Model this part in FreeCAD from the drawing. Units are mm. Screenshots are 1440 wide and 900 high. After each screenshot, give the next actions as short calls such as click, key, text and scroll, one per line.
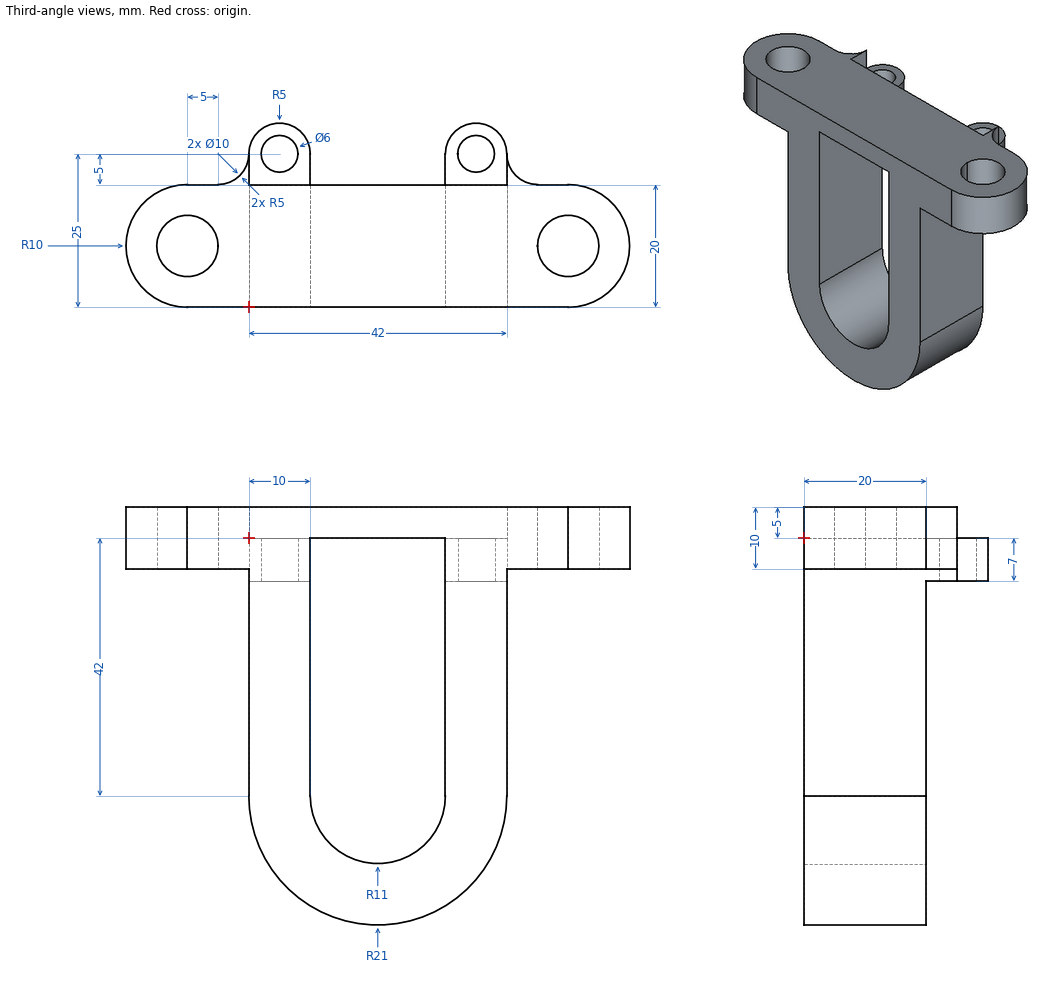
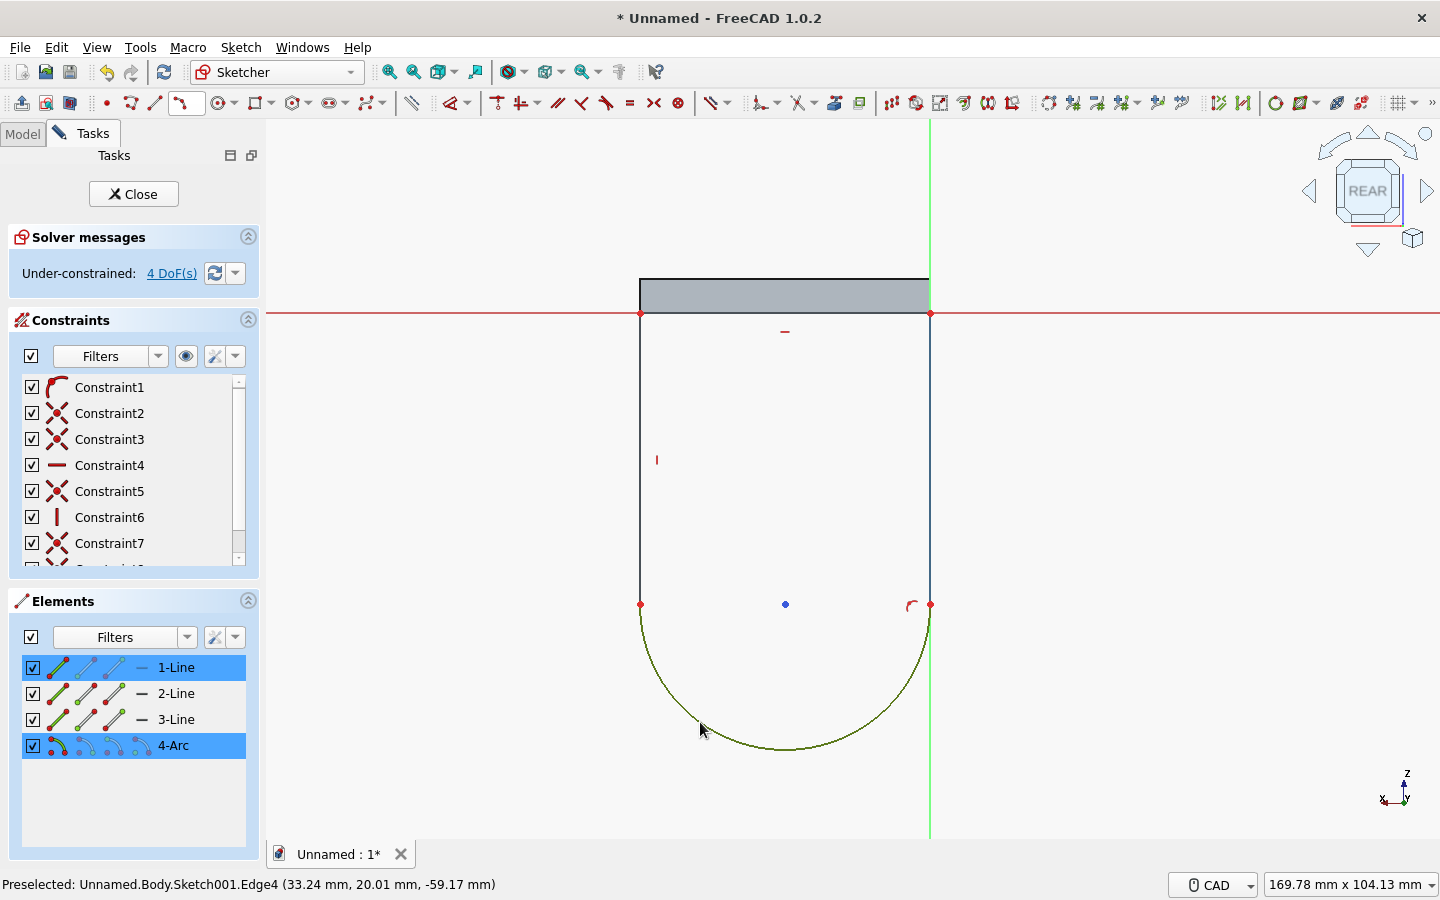
click(606, 104)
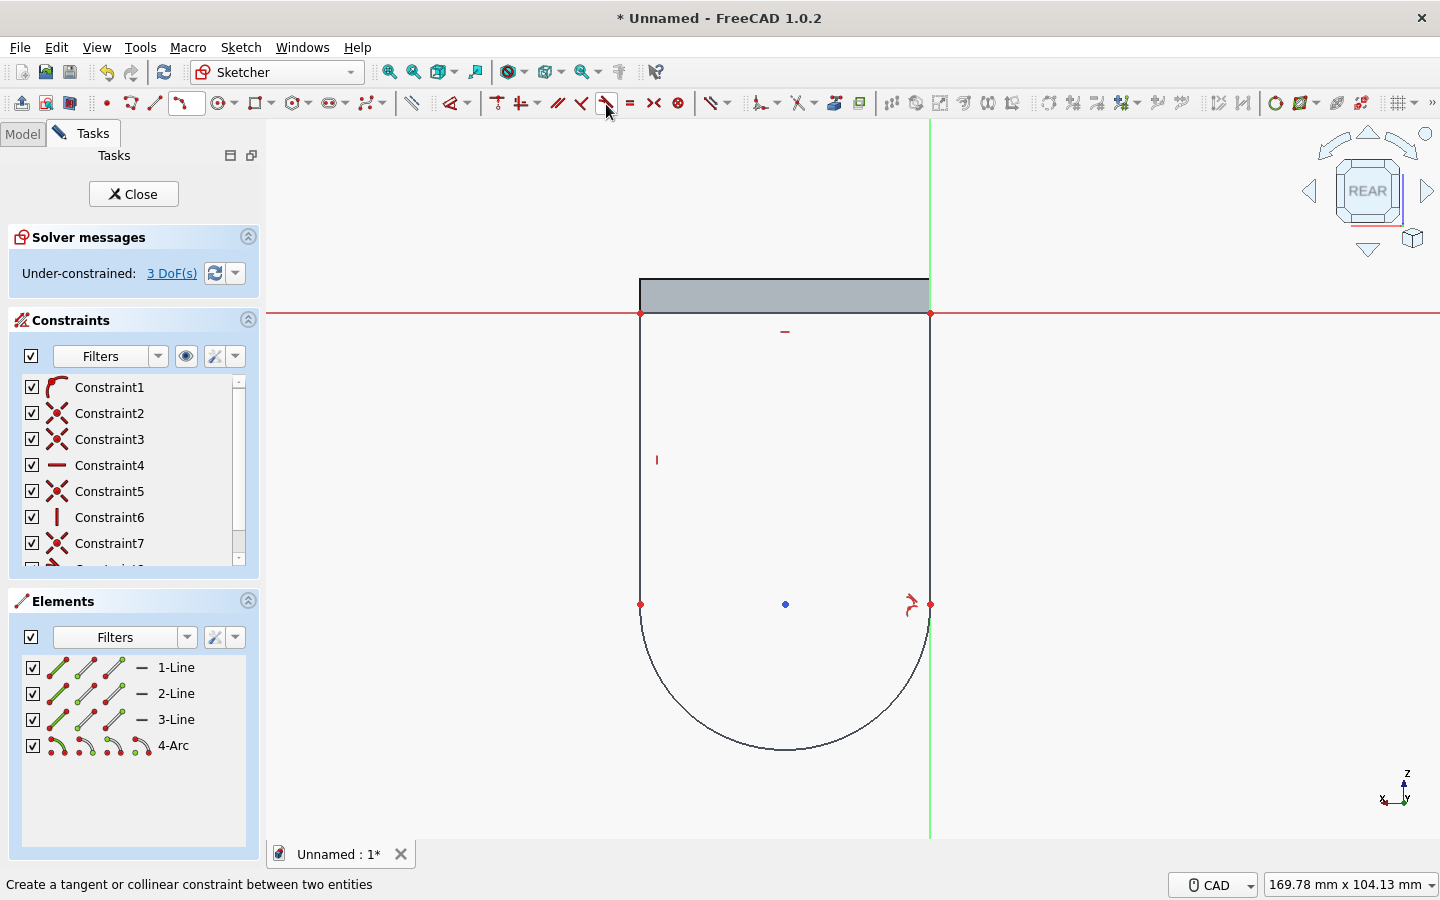
click(640, 401)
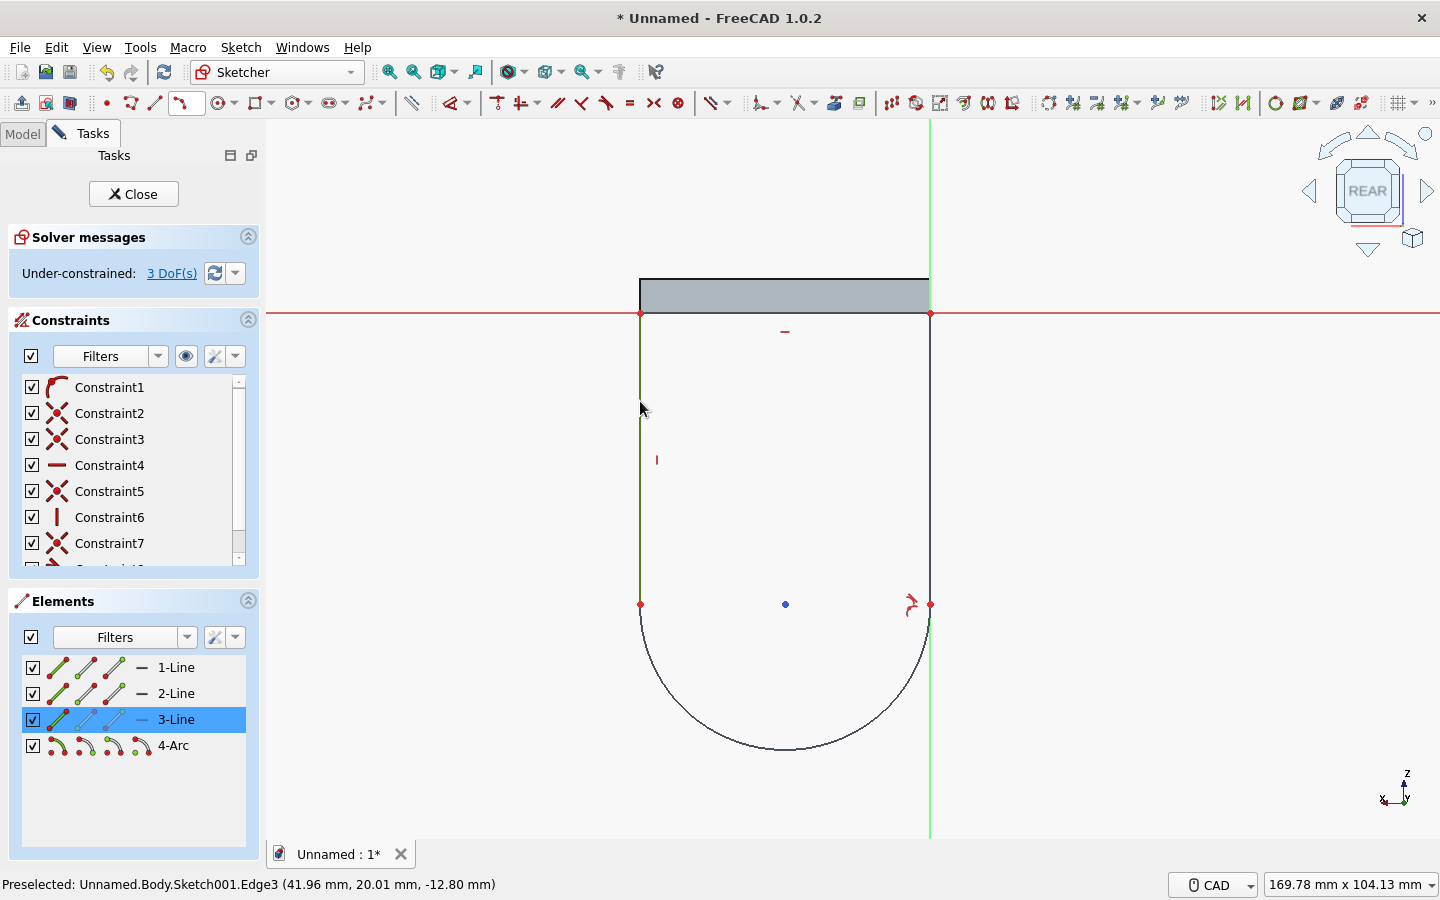
click(700, 722)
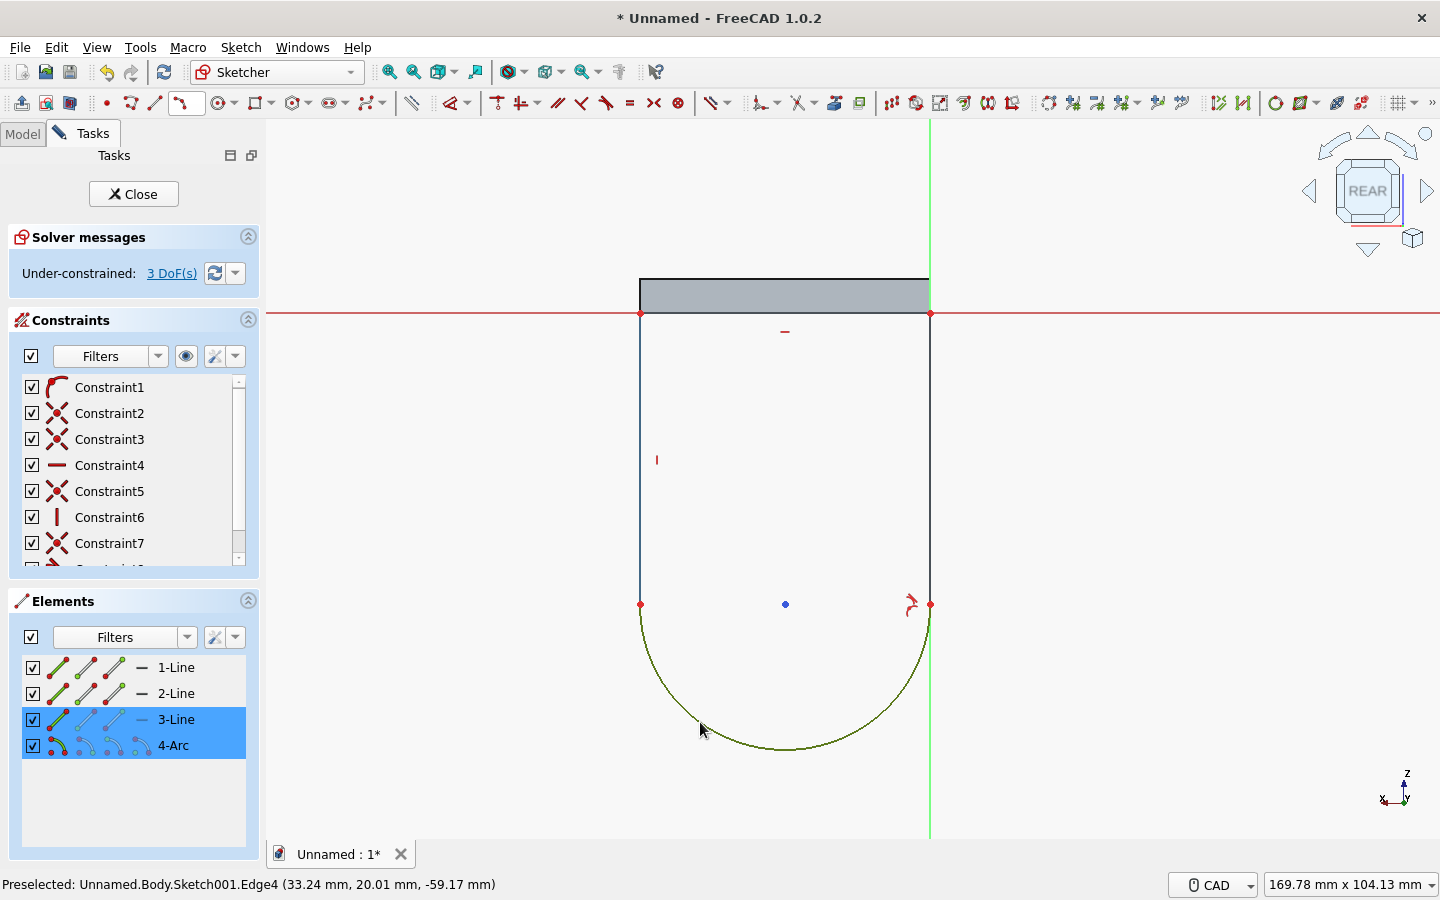
click(606, 104)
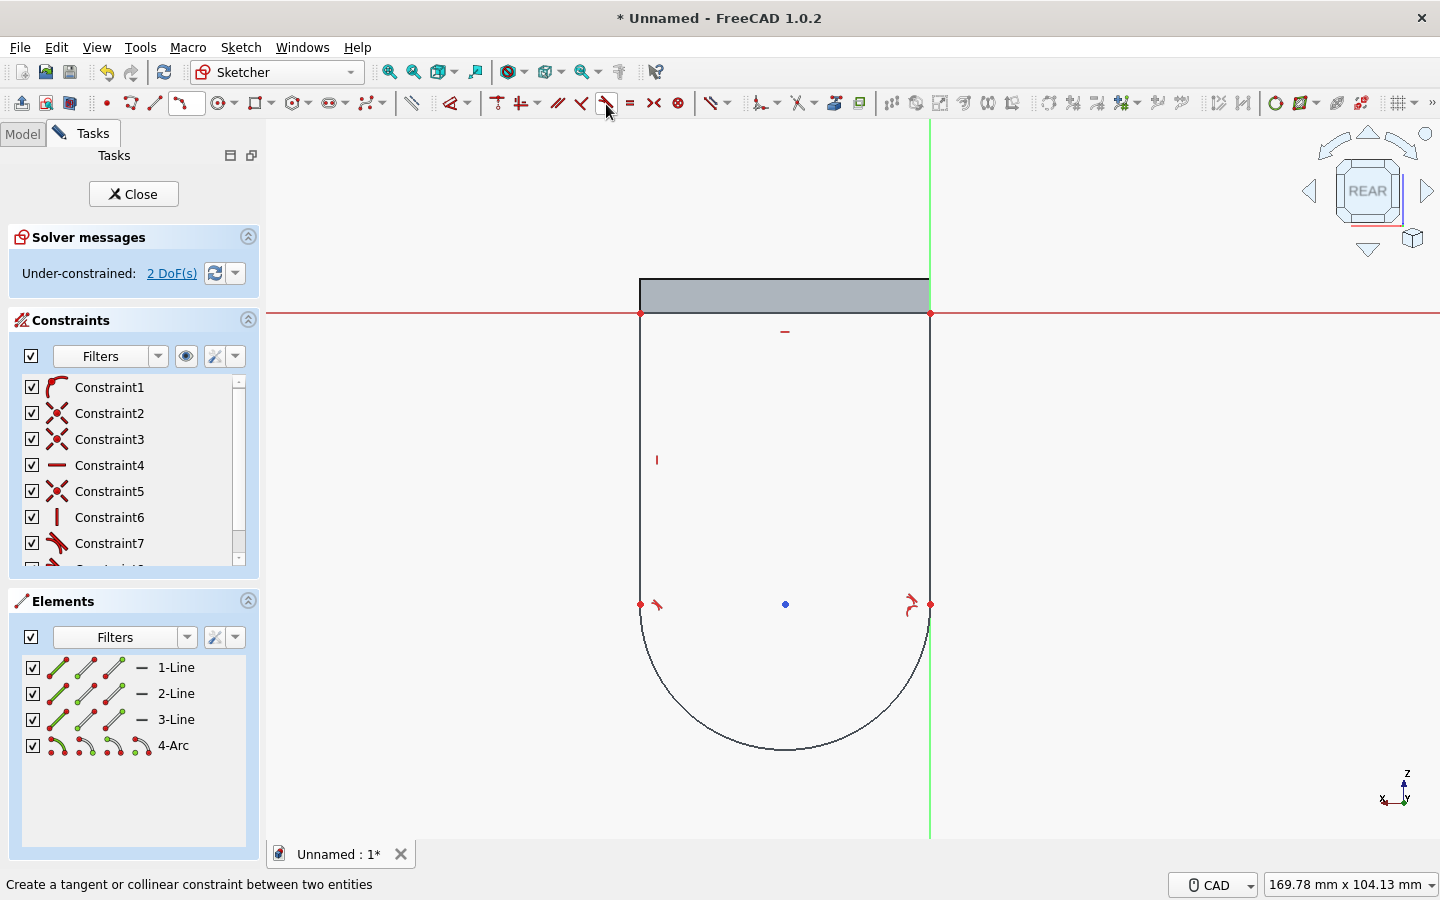
click(450, 104)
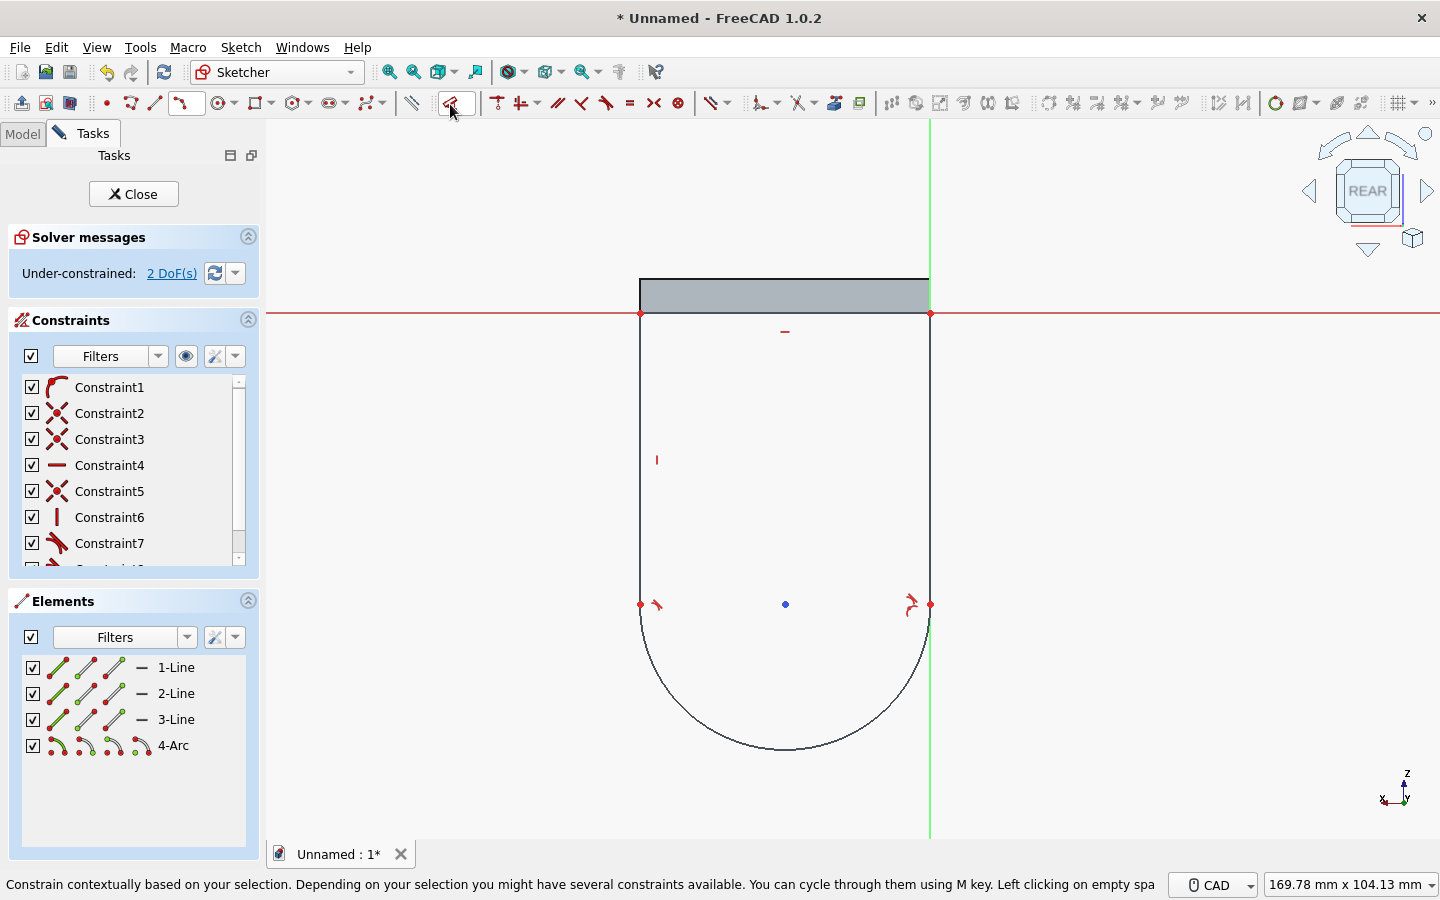
click(700, 722)
click(681, 748)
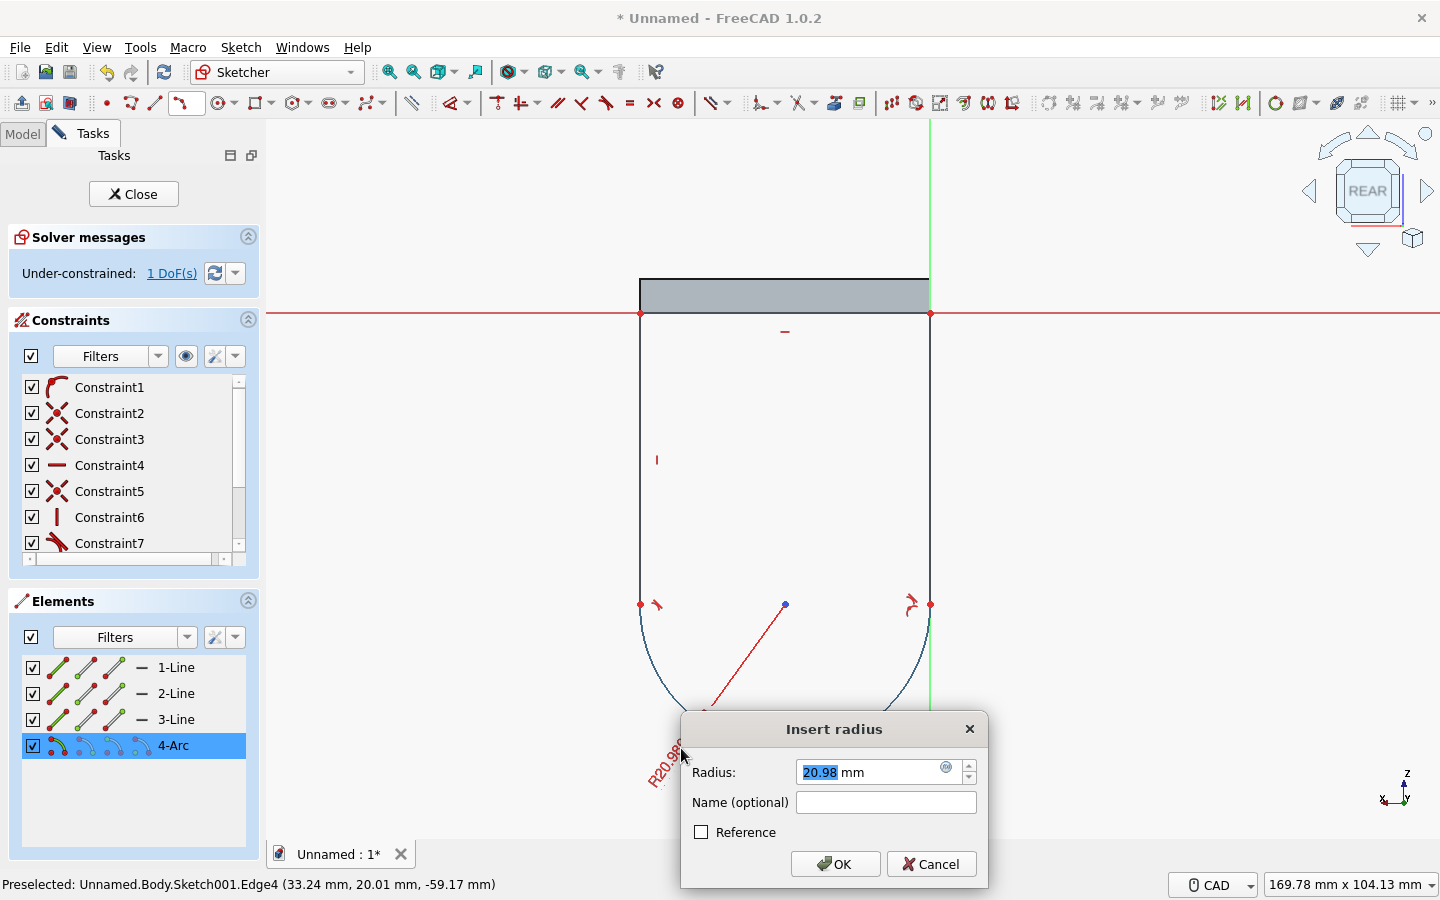
text(21)
key(Return)